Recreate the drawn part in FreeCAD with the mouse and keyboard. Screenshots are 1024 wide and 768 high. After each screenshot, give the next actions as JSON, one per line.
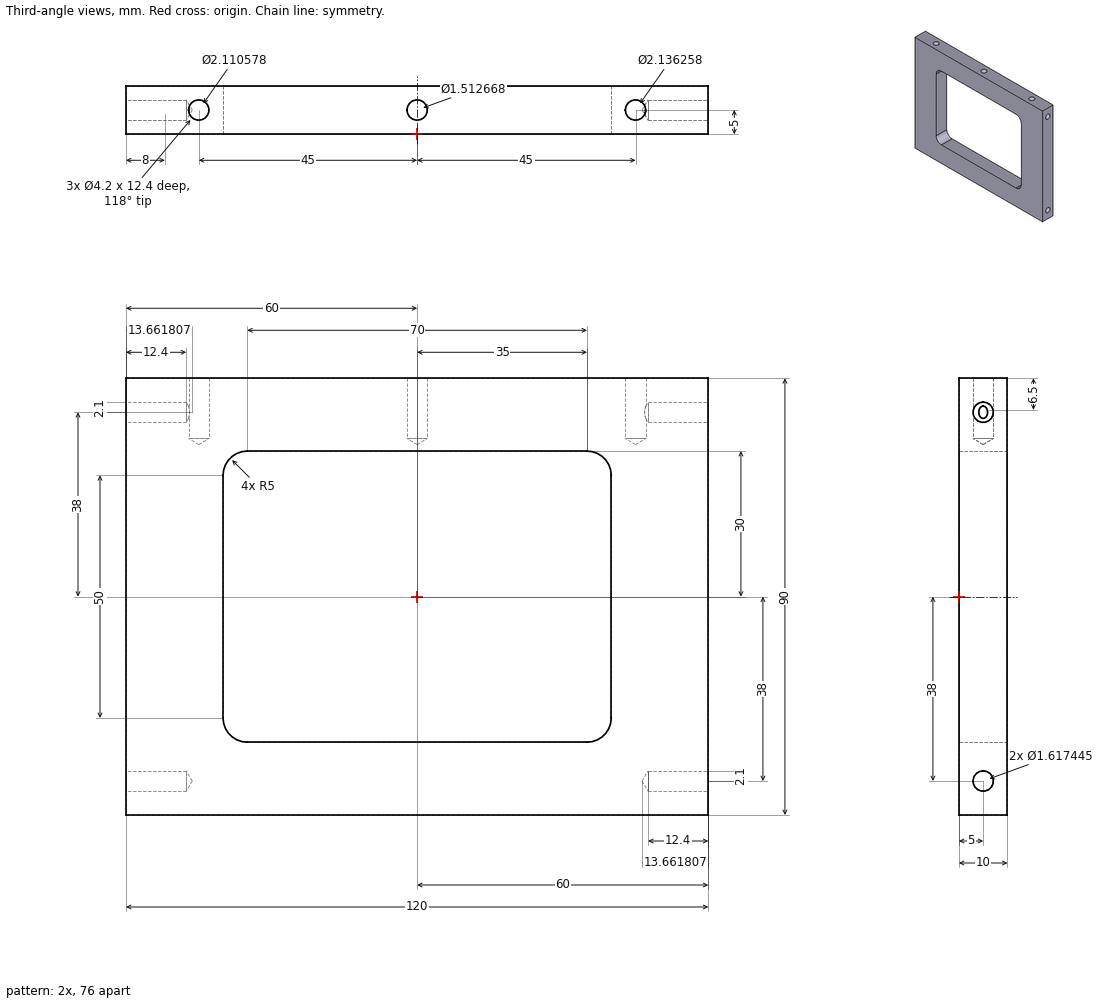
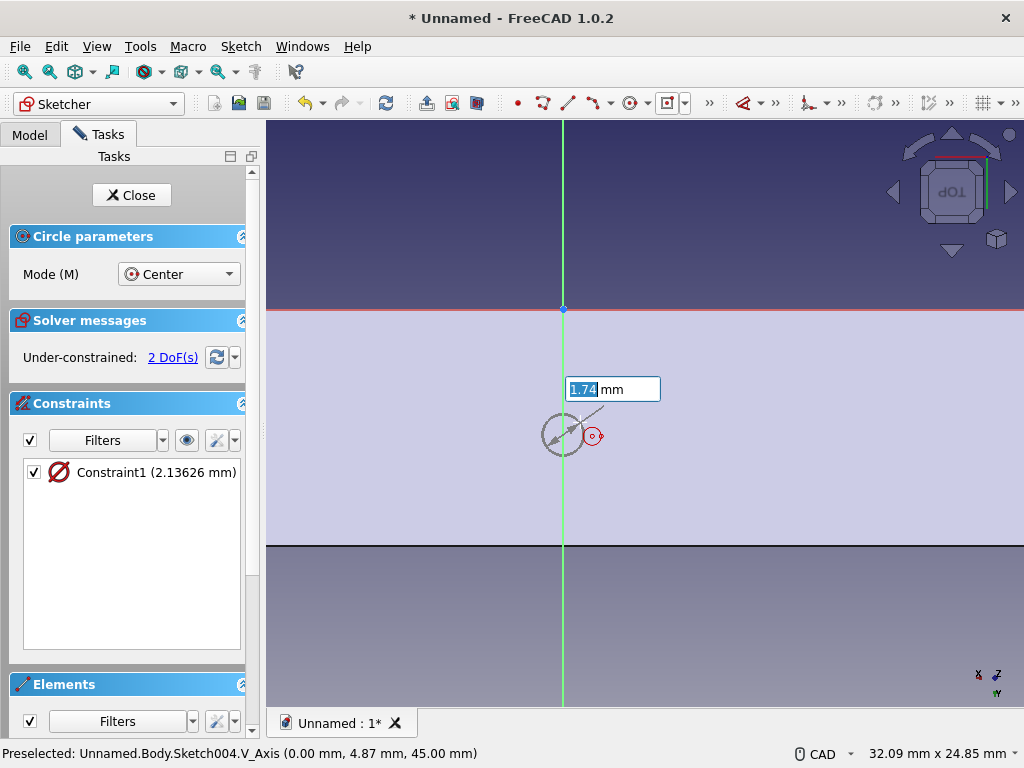
{"action": "type", "text": "1.512668"}
{"action": "key", "text": "Return"}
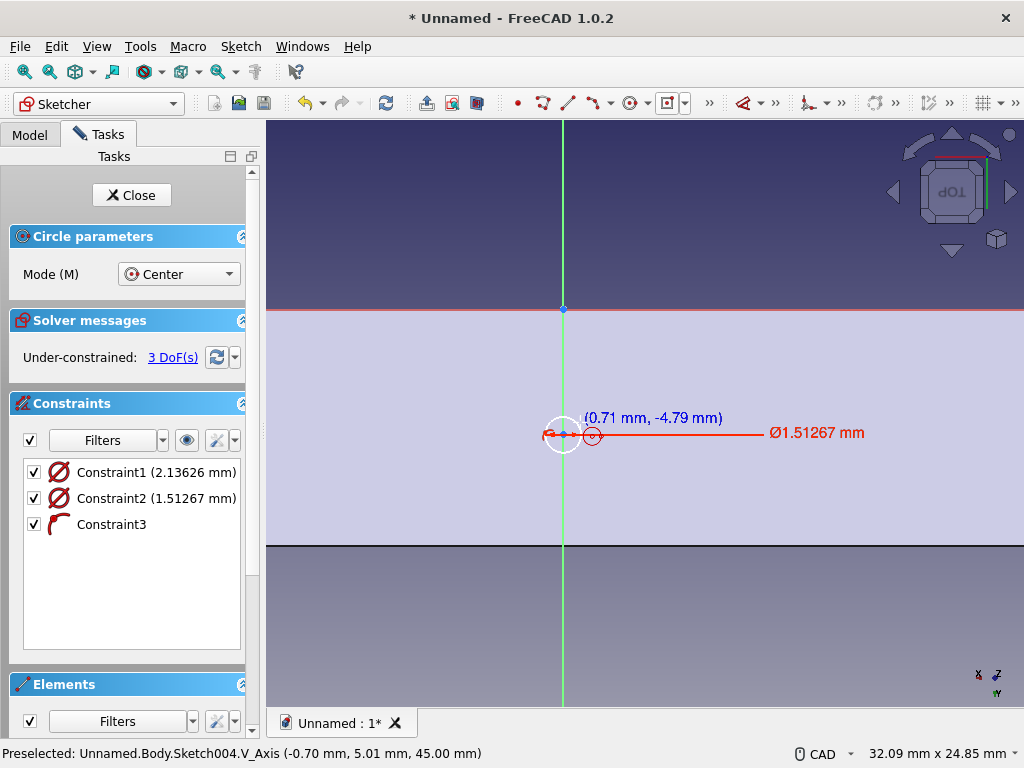
{"action": "scroll", "coordinate": [580, 422], "scroll_direction": "down", "scroll_amount": 8}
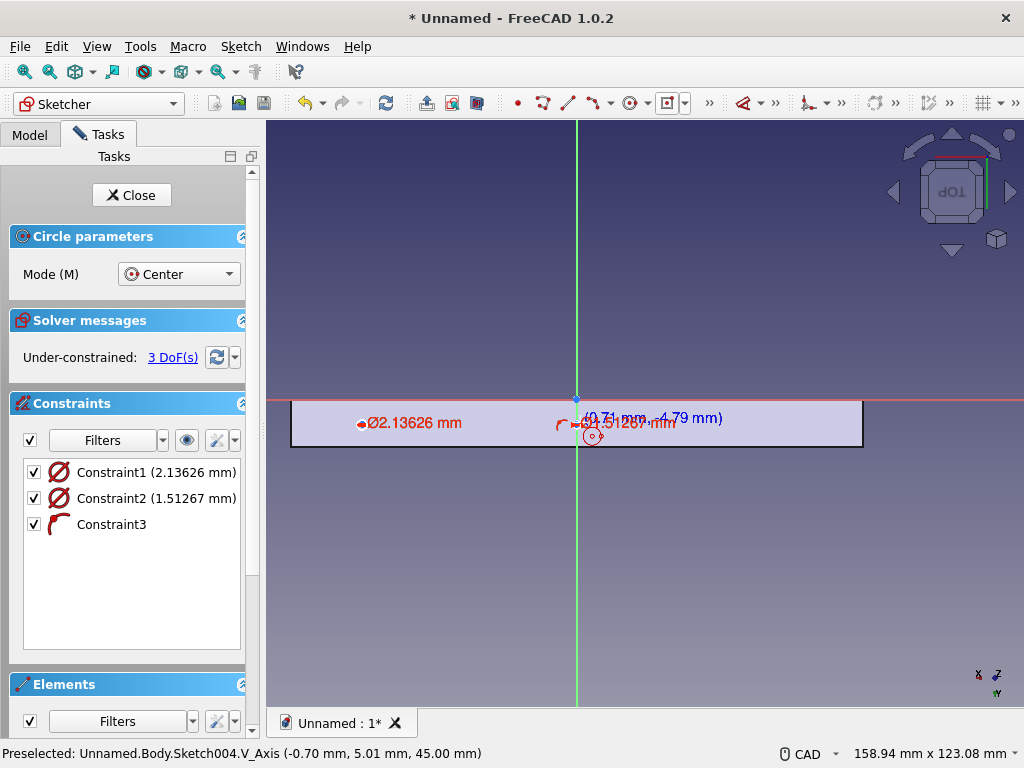
{"action": "scroll", "coordinate": [792, 424], "scroll_direction": "up", "scroll_amount": 8}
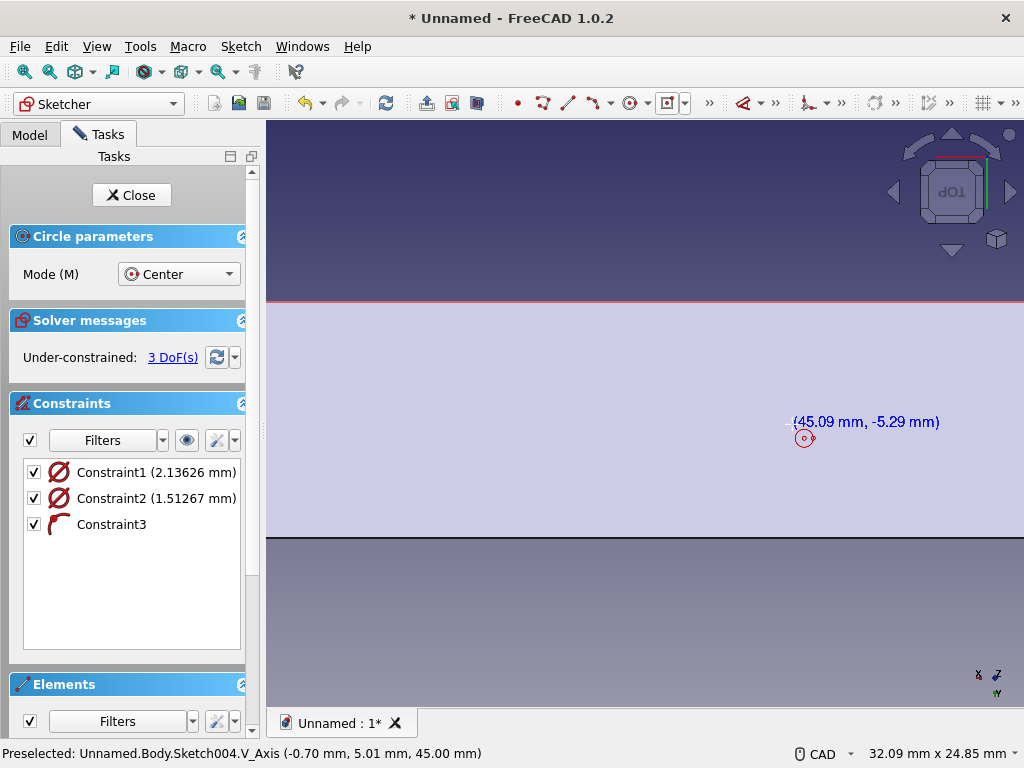
{"action": "scroll", "coordinate": [792, 424], "scroll_direction": "down", "scroll_amount": 8}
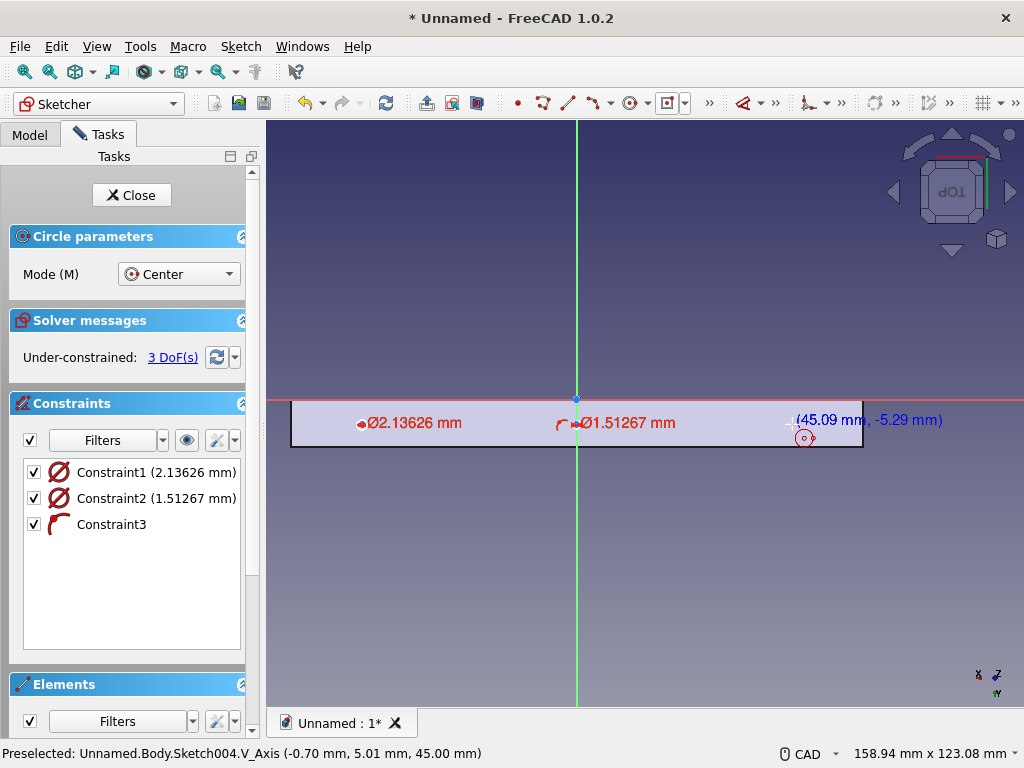
{"action": "left_click", "coordinate": [792, 424]}
{"action": "mouse_move", "coordinate": [795, 420]}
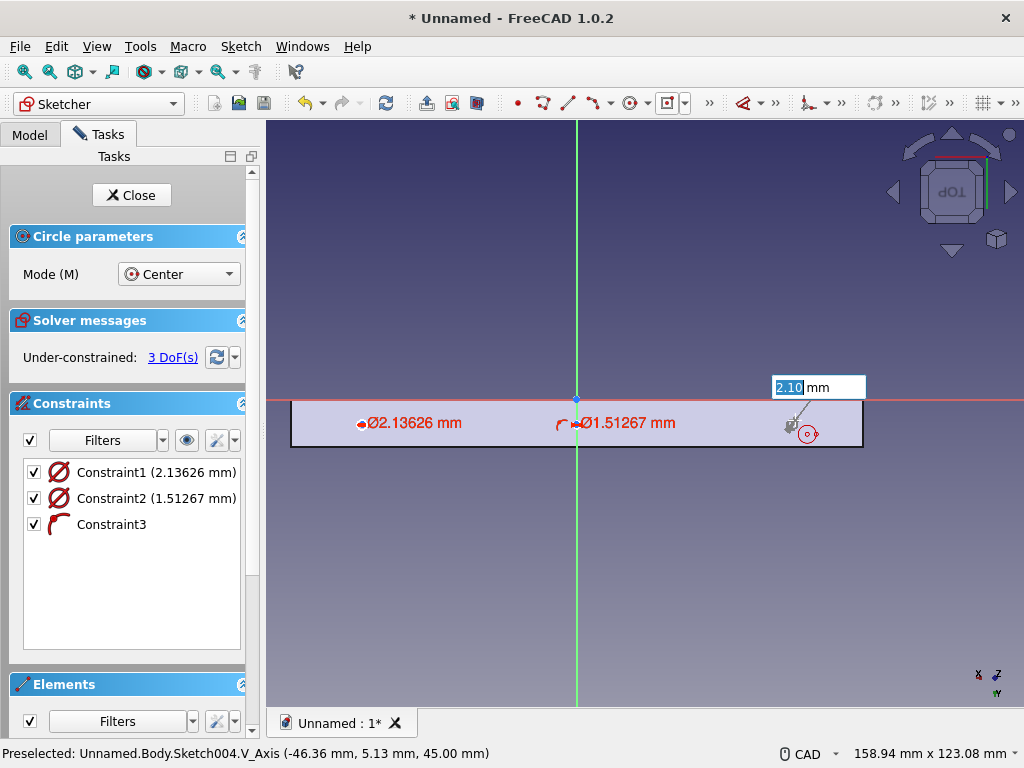
{"action": "type", "text": "2.110578"}
{"action": "key", "text": "Return"}
{"action": "key", "text": "Escape"}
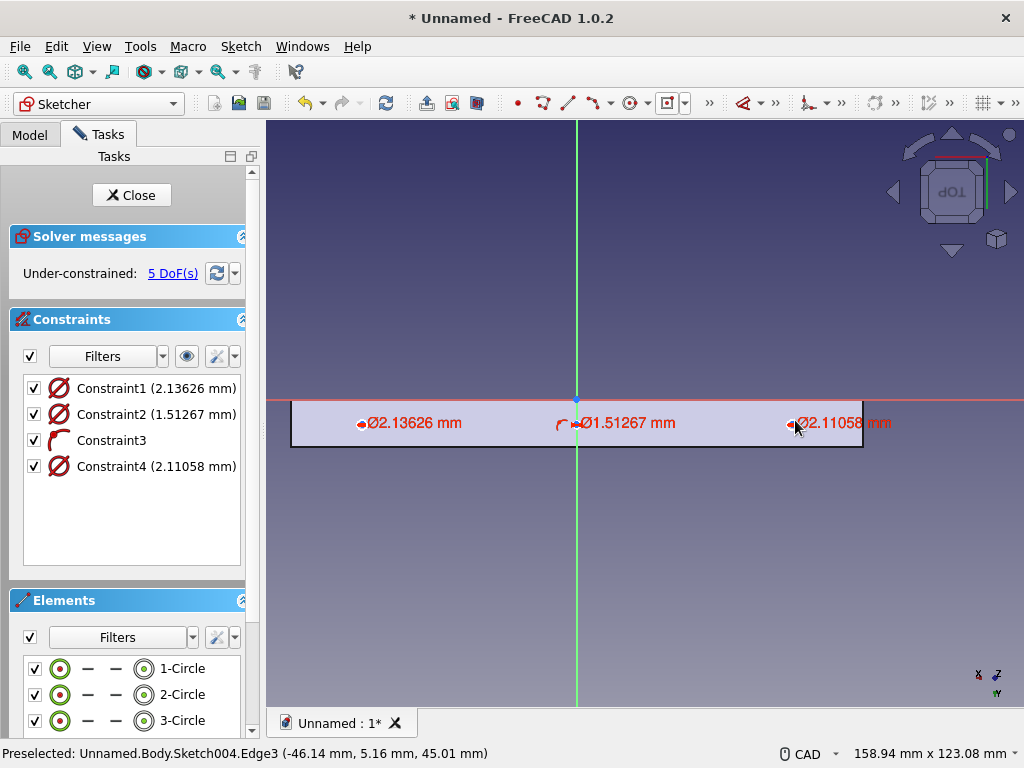
{"action": "left_click", "coordinate": [362, 425]}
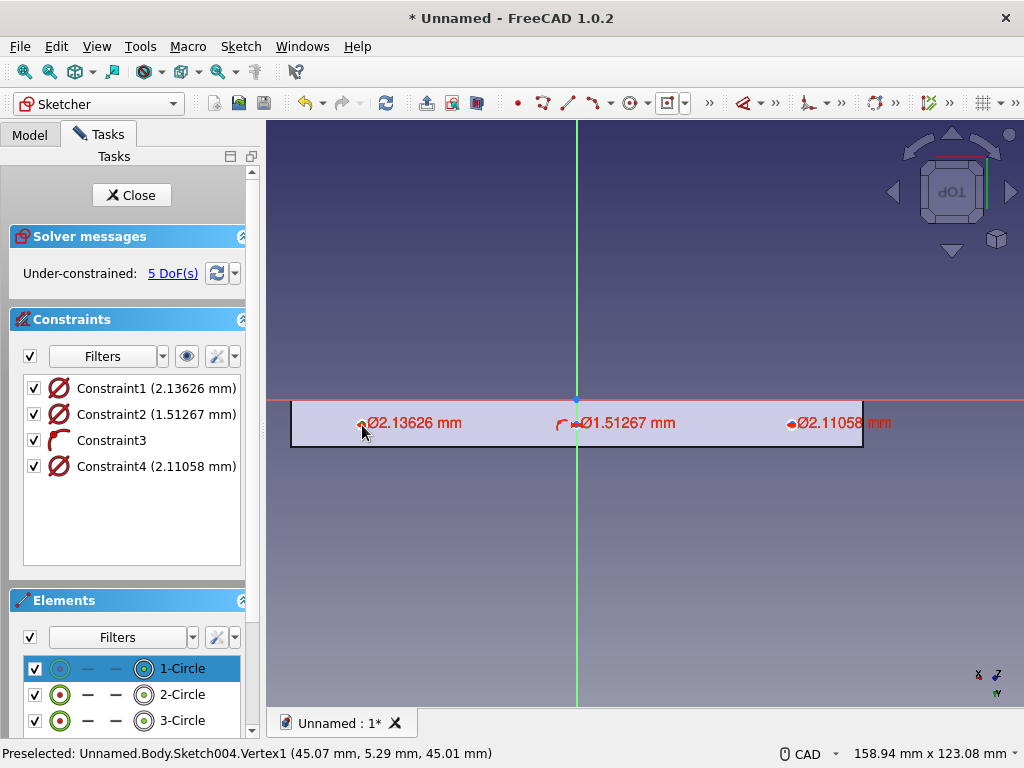
{"action": "left_click", "coordinate": [792, 425]}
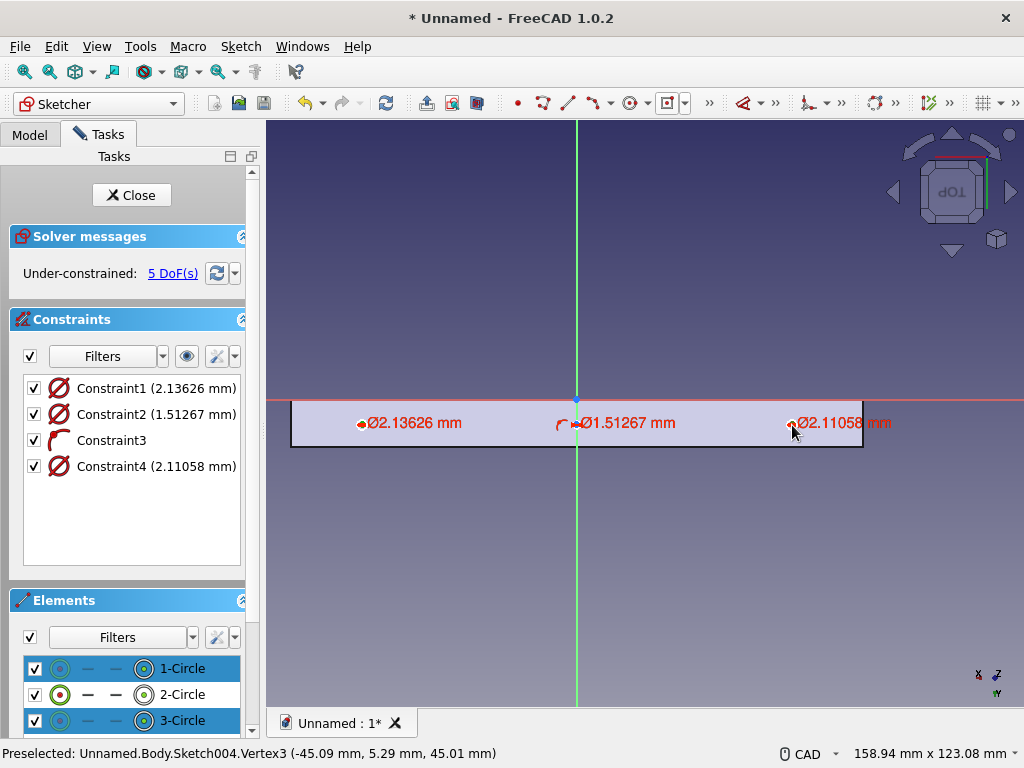
{"action": "left_click", "coordinate": [577, 641]}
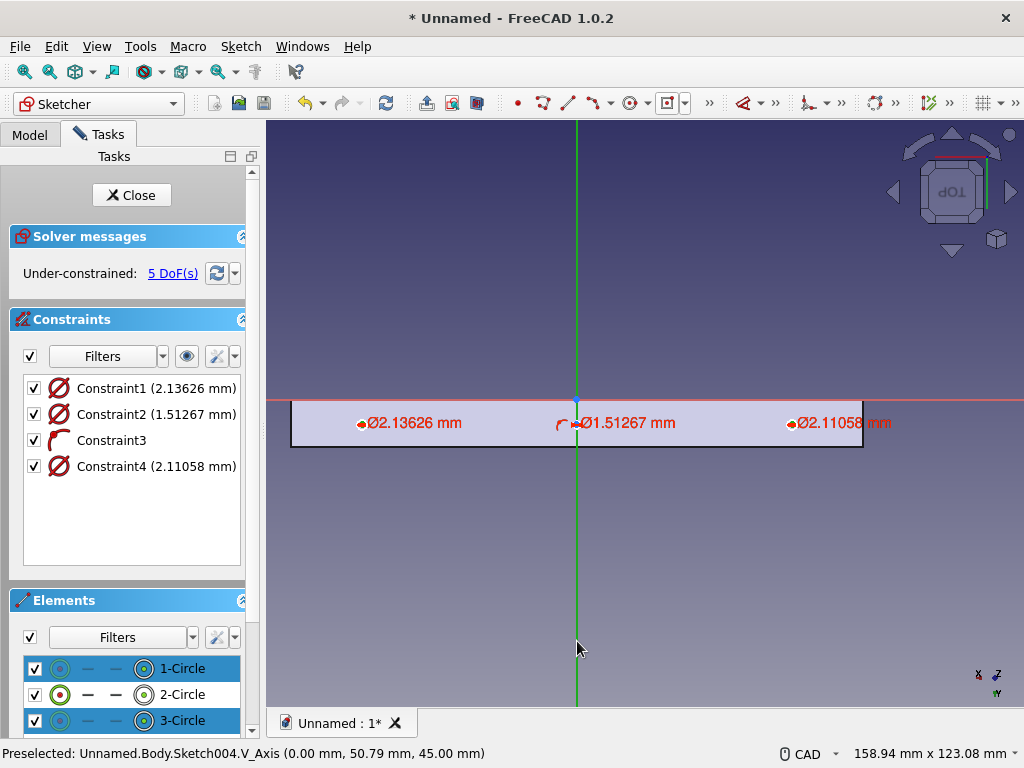
{"action": "key", "text": "s"}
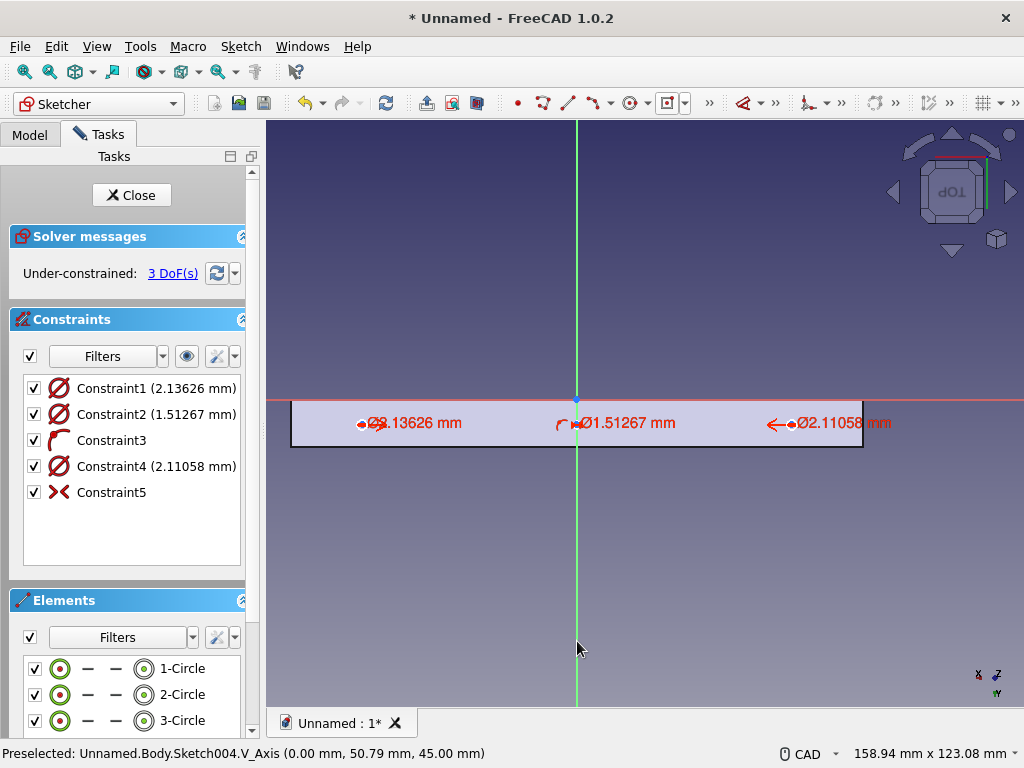
{"action": "left_click", "coordinate": [742, 104]}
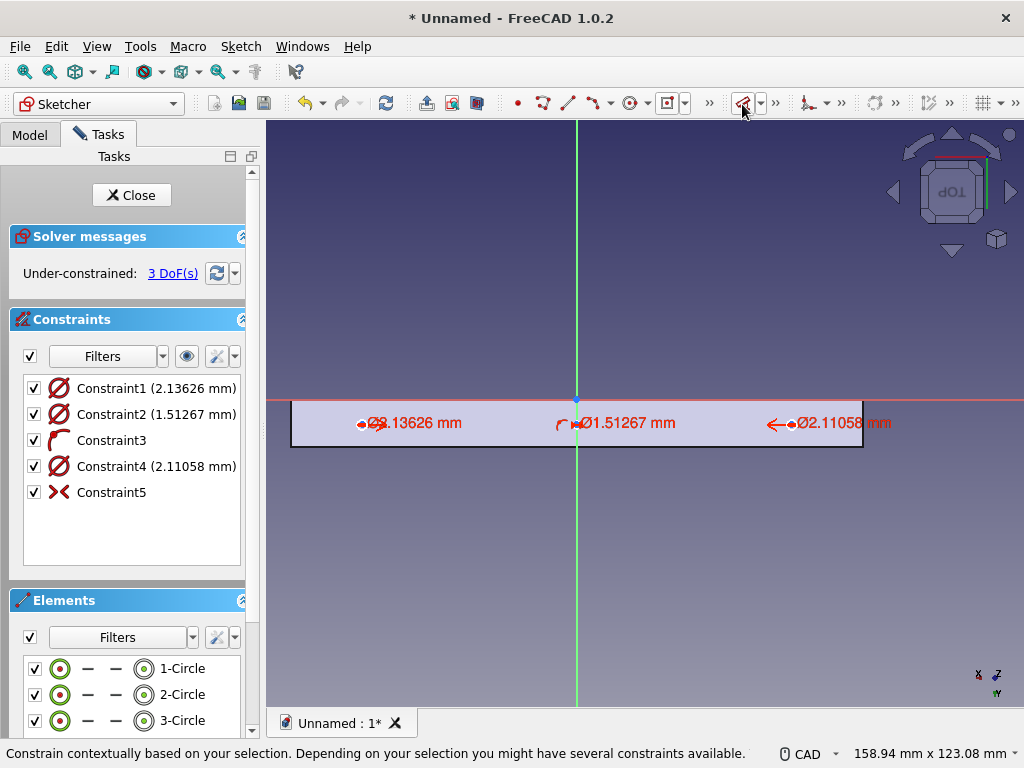
{"action": "scroll", "coordinate": [362, 425], "scroll_direction": "up", "scroll_amount": 3}